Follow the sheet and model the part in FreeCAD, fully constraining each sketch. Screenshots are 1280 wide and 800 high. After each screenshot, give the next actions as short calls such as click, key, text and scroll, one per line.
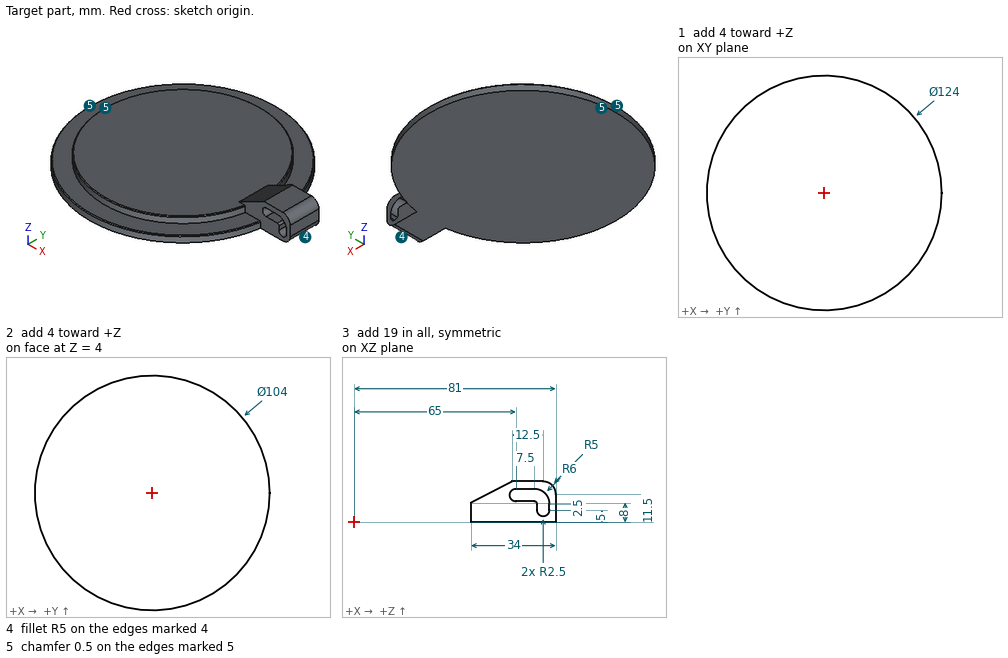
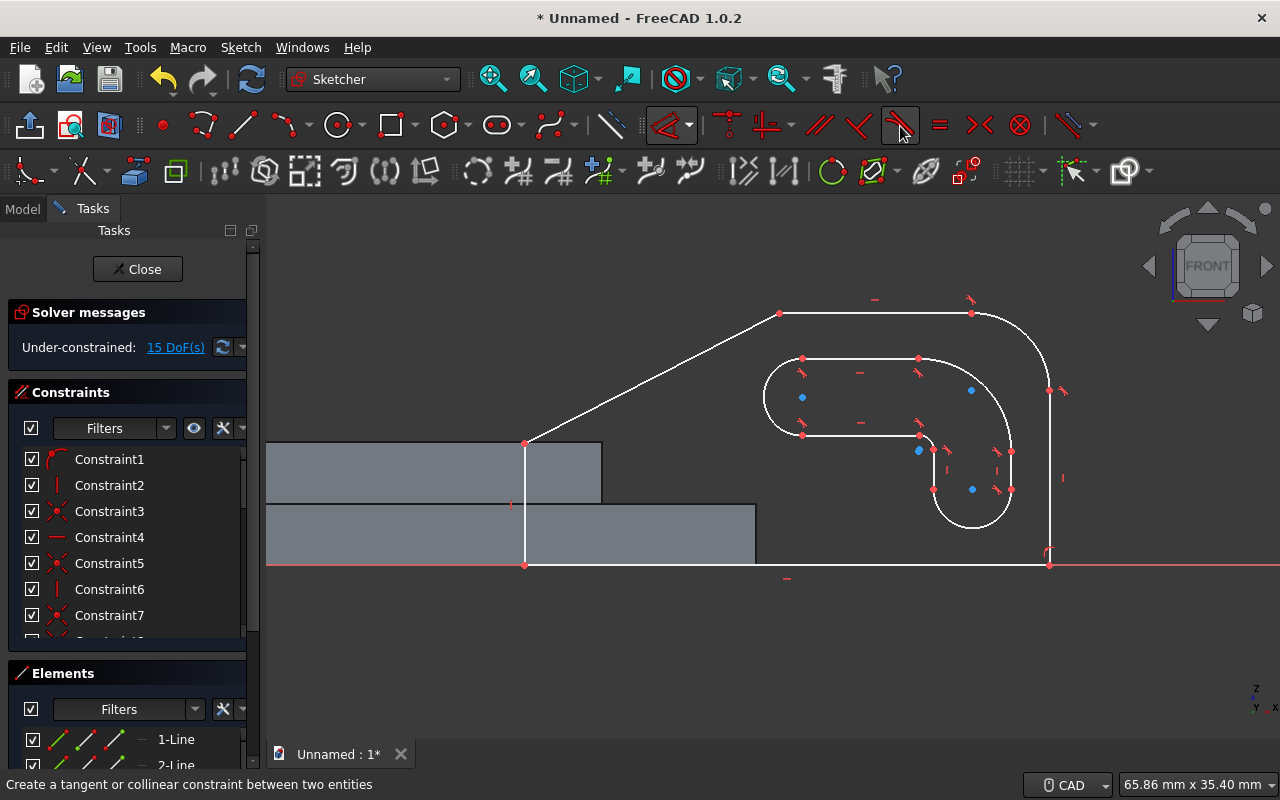
click(934, 462)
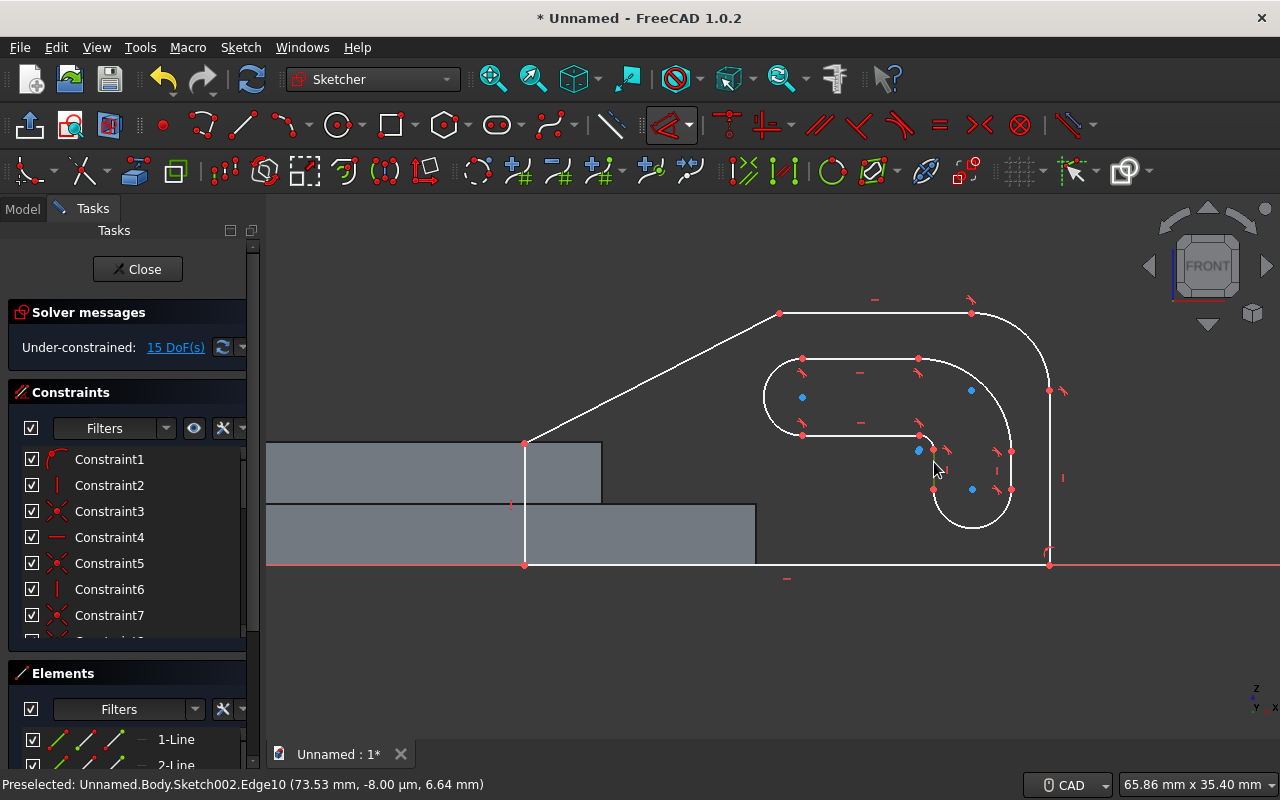
click(950, 521)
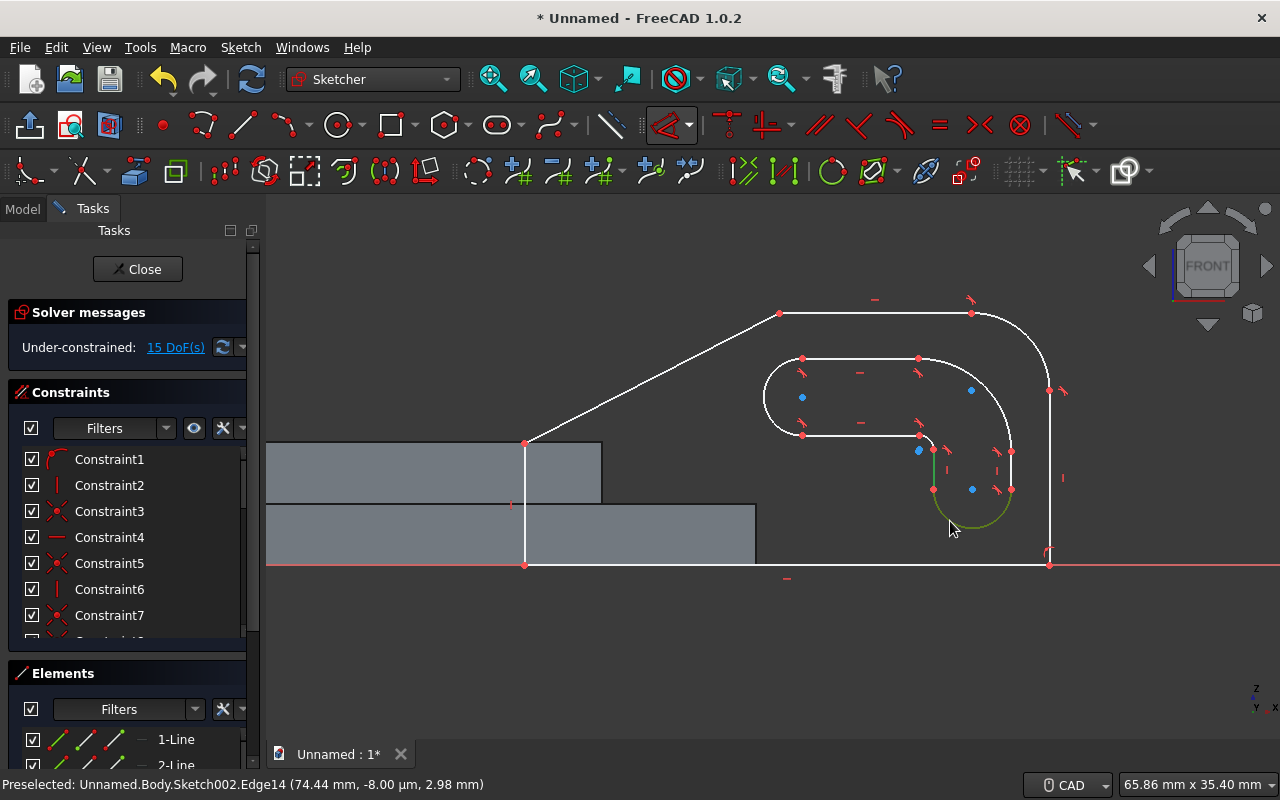
click(900, 126)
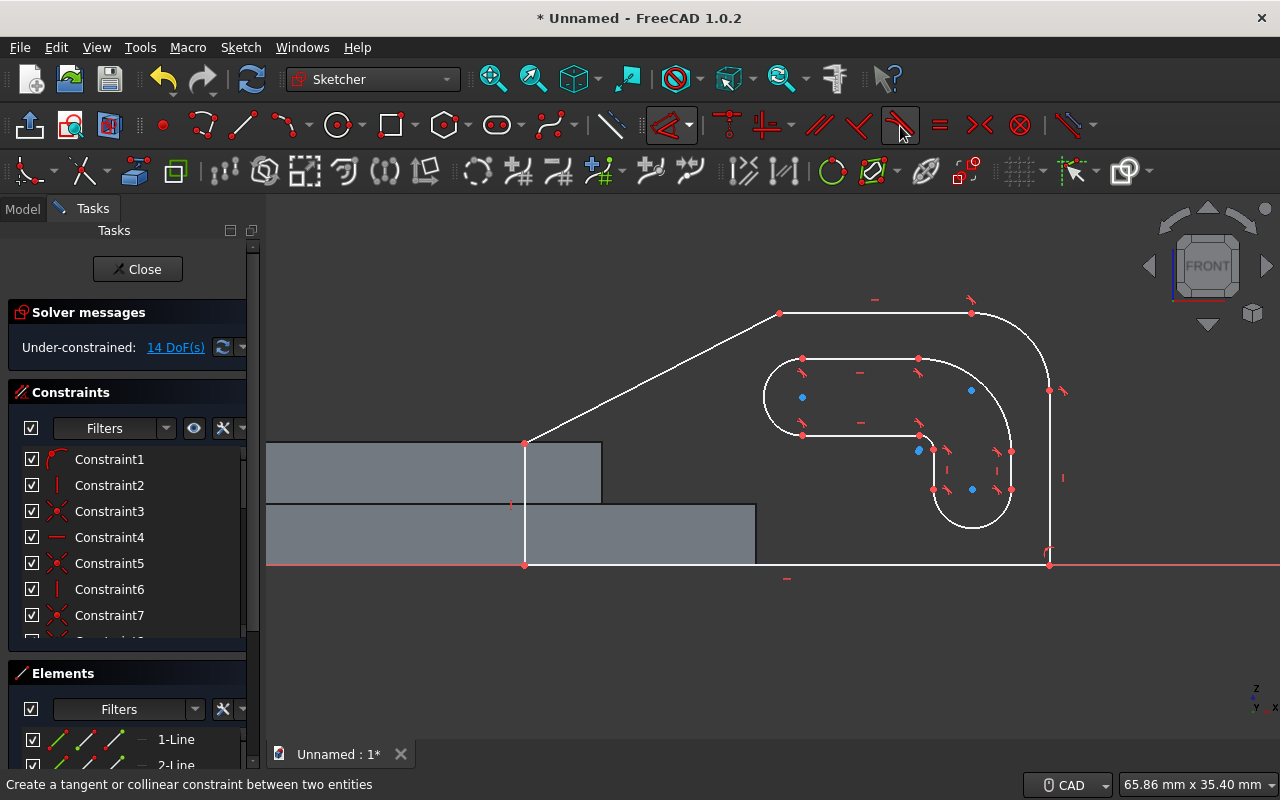
click(1001, 409)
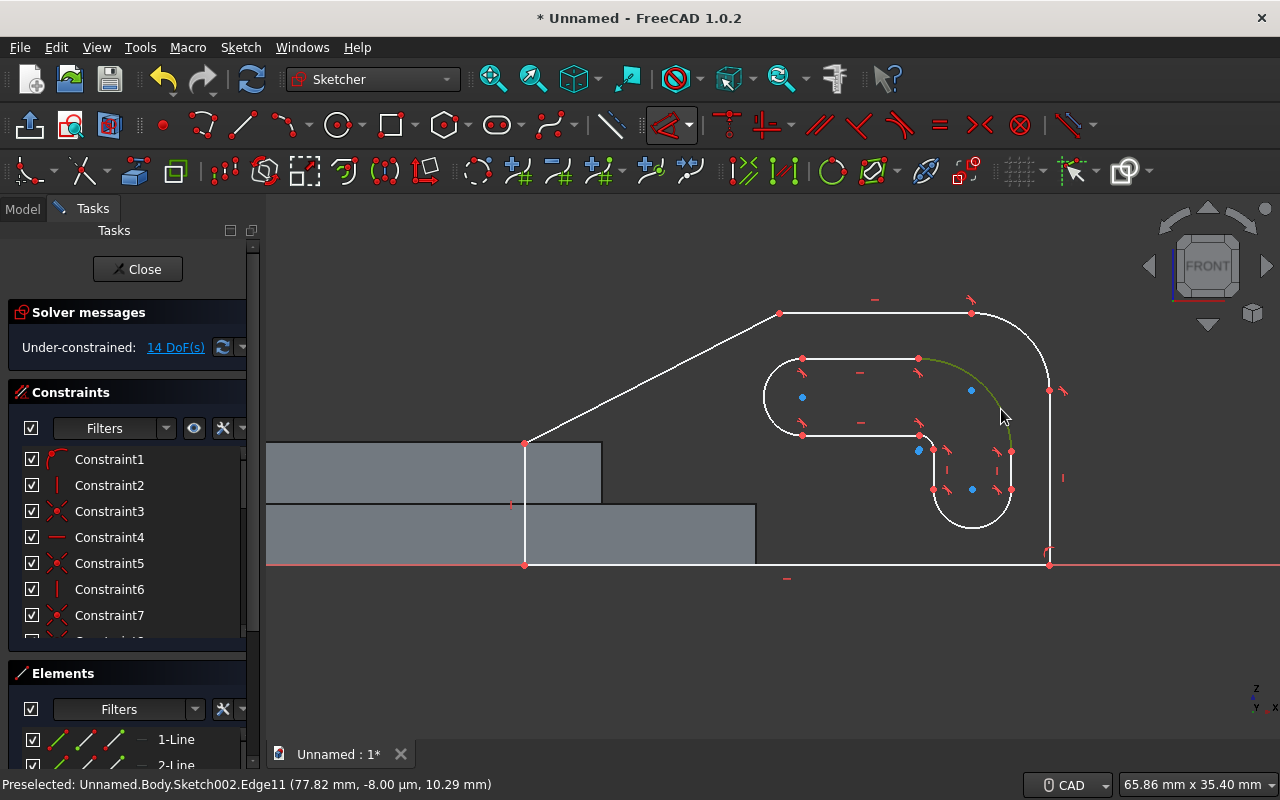
scroll(930, 440, up, 2)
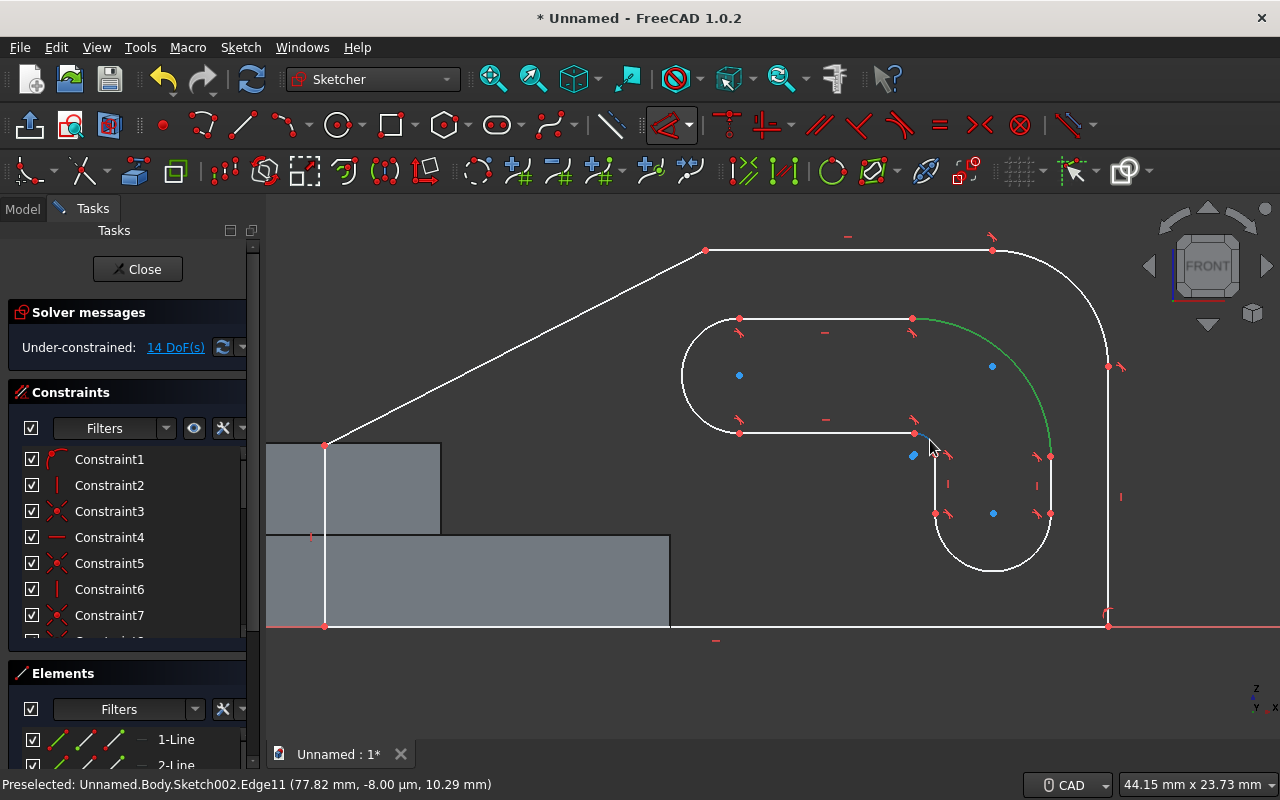
click(929, 439)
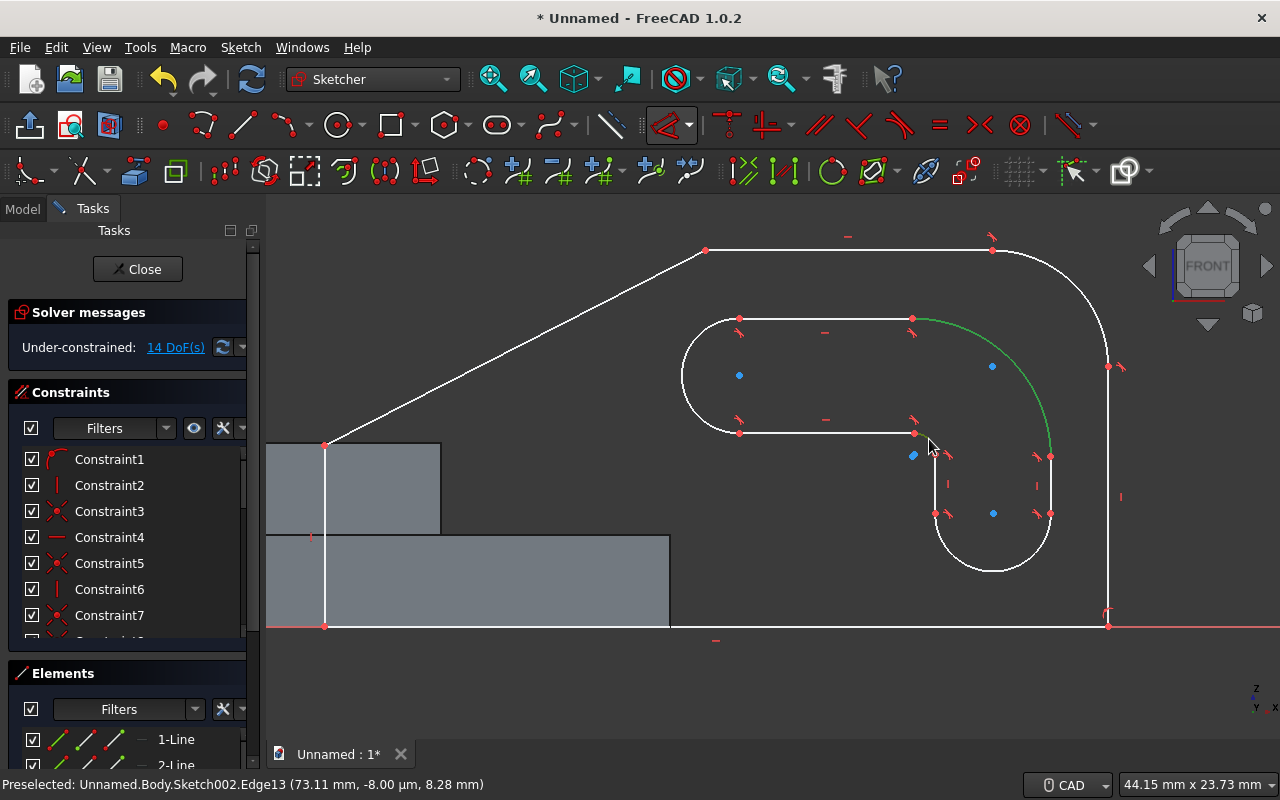
click(728, 126)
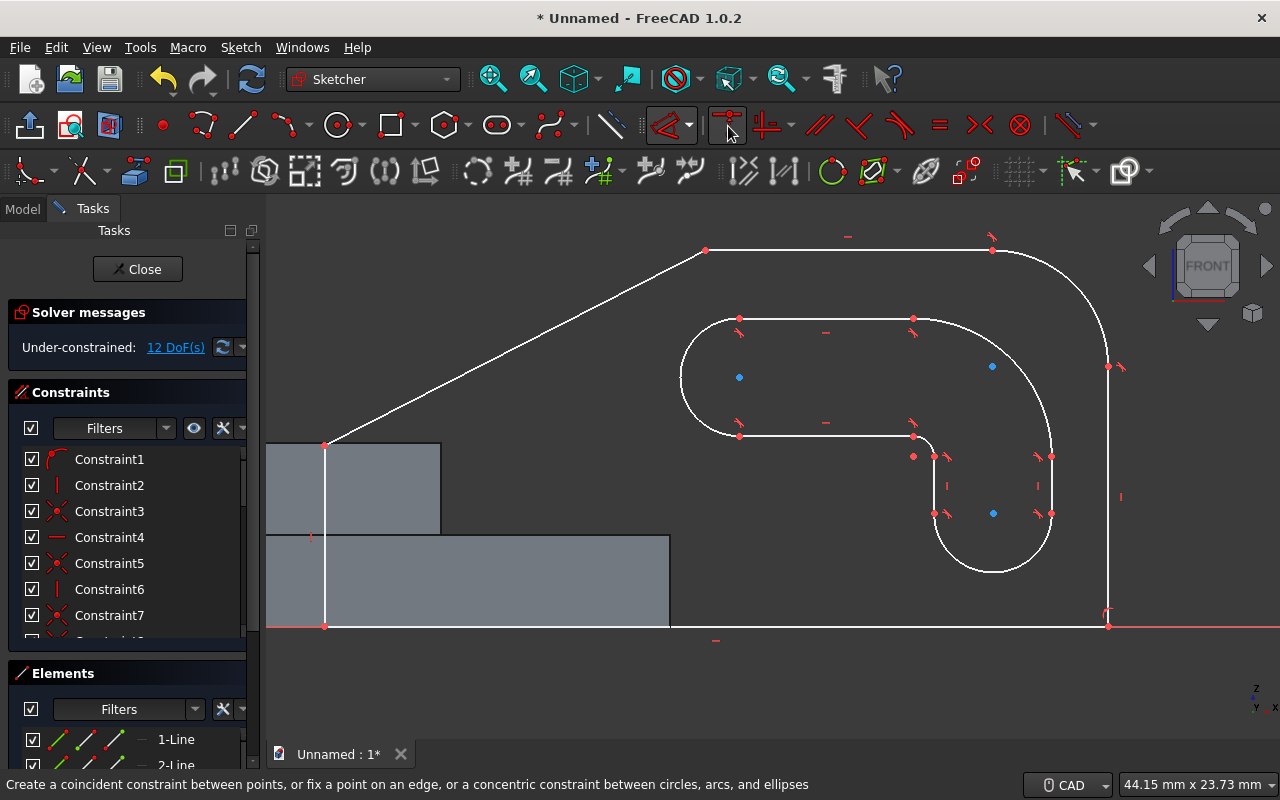
click(1095, 314)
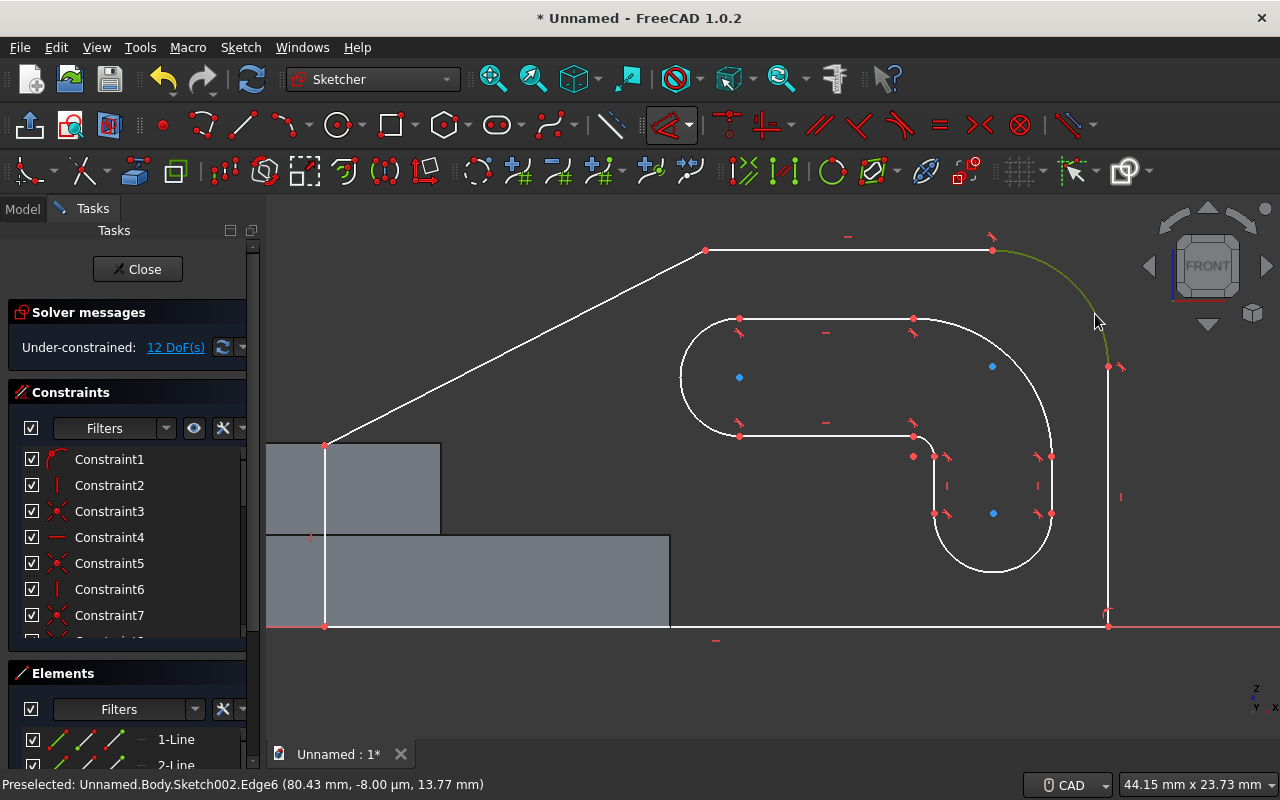
key(k)
key(r)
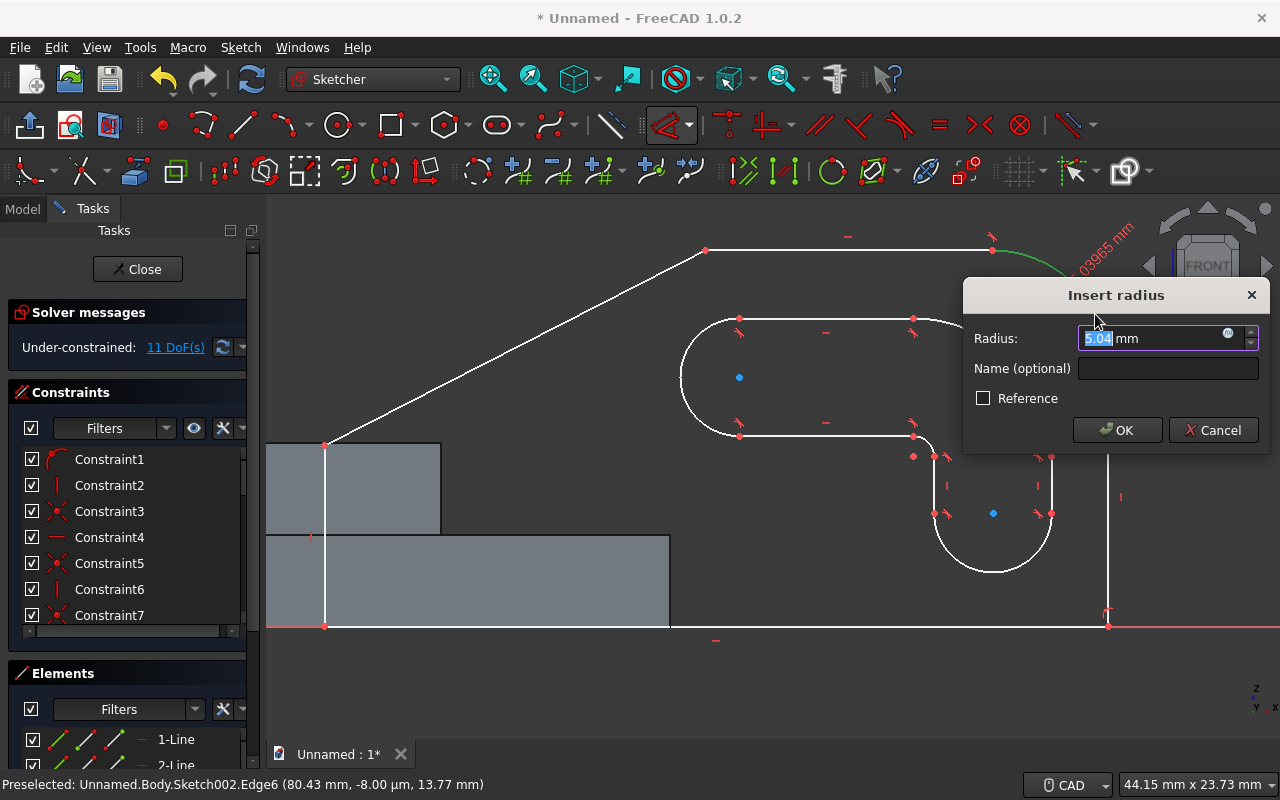
text(5)
key(Return)